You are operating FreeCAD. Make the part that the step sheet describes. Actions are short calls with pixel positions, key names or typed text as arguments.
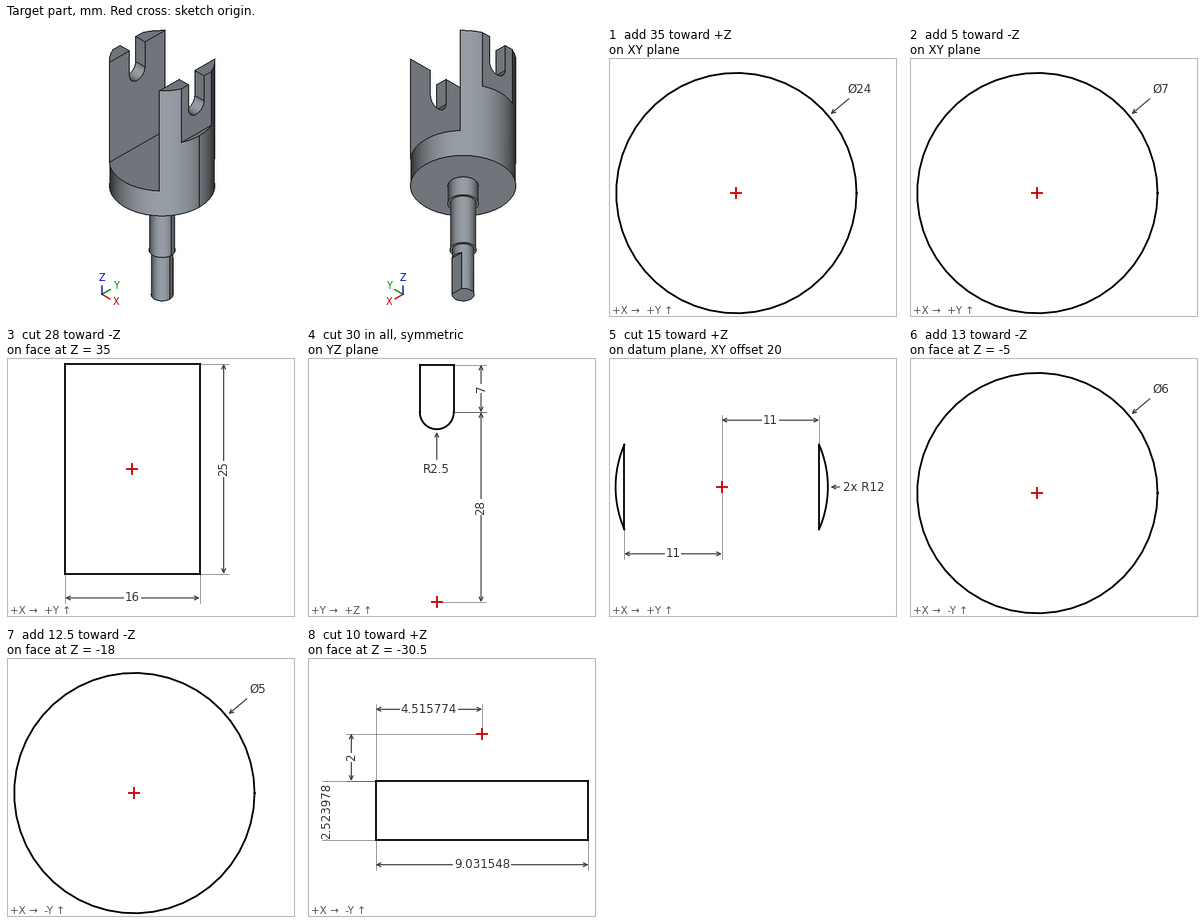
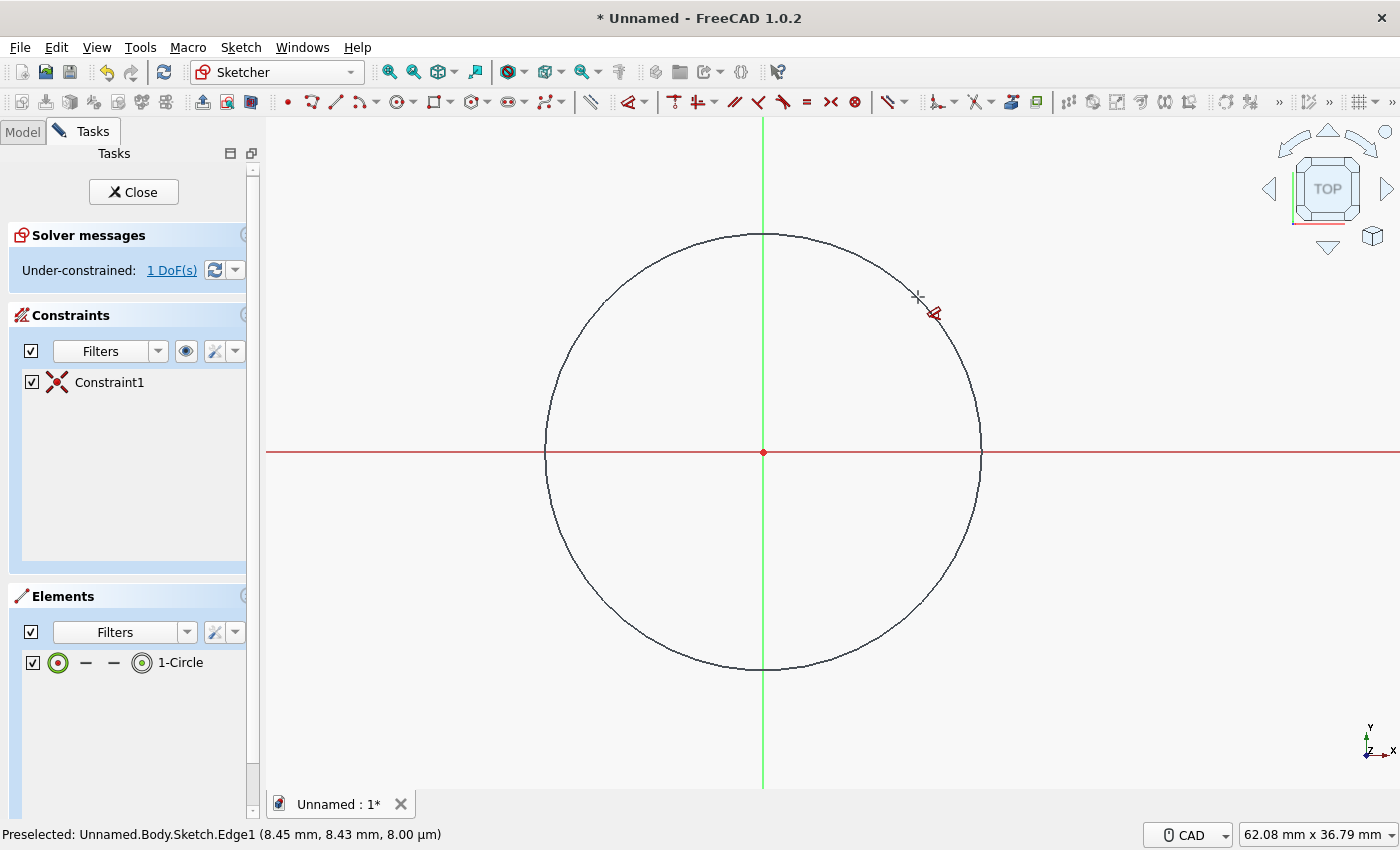
click(917, 297)
click(940, 274)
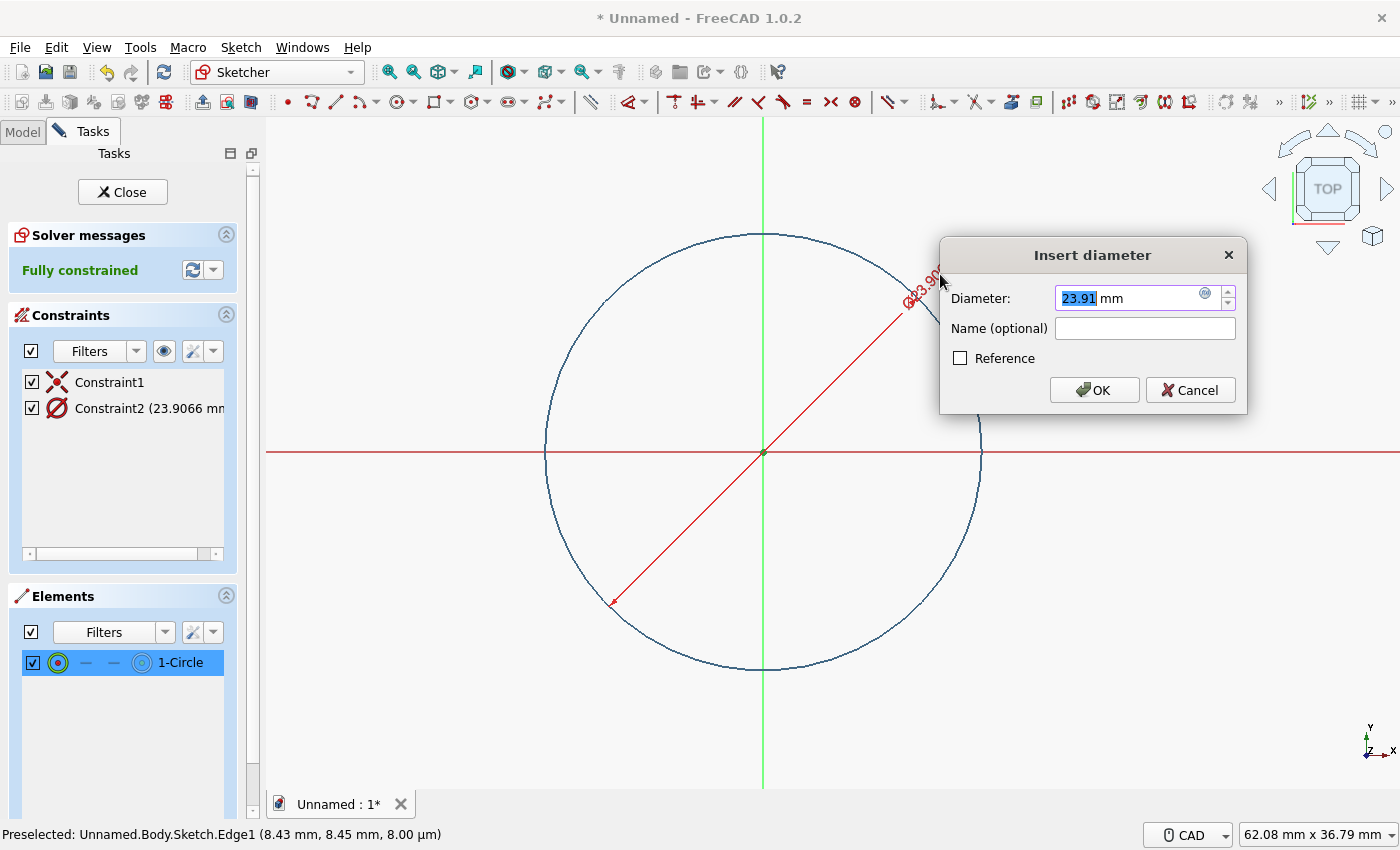
text(24)
key(Return)
key(Escape)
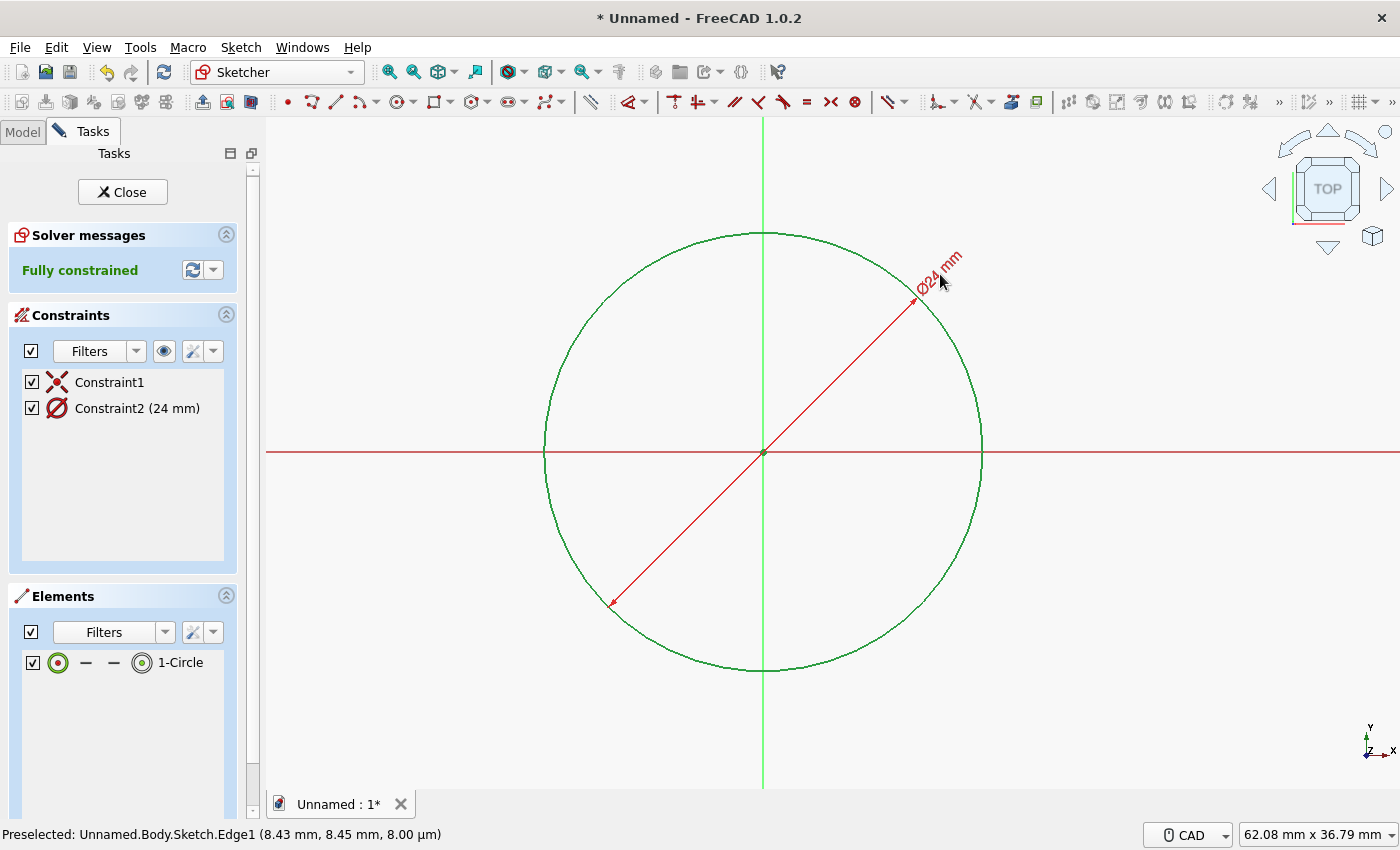
click(123, 192)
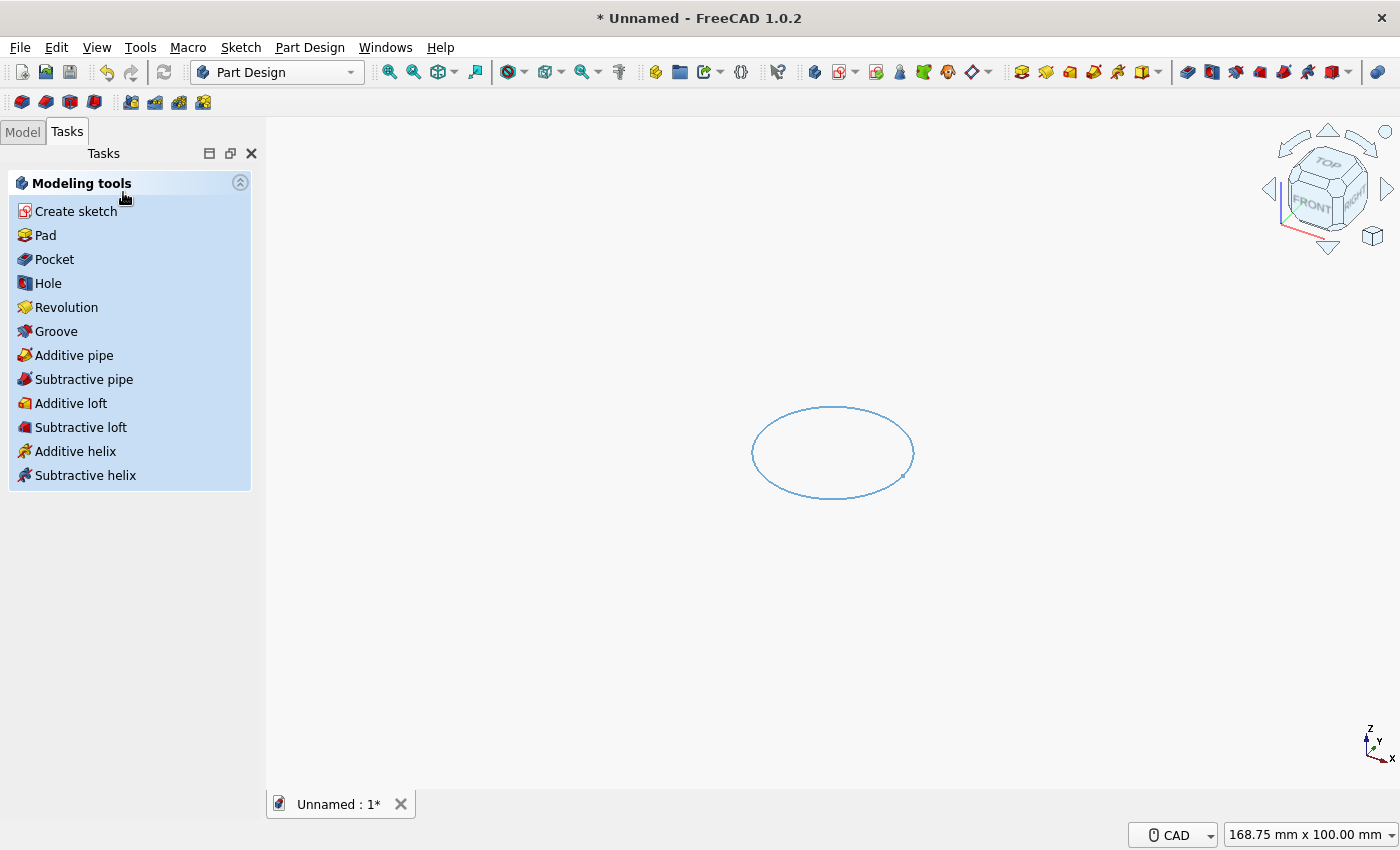
click(1022, 72)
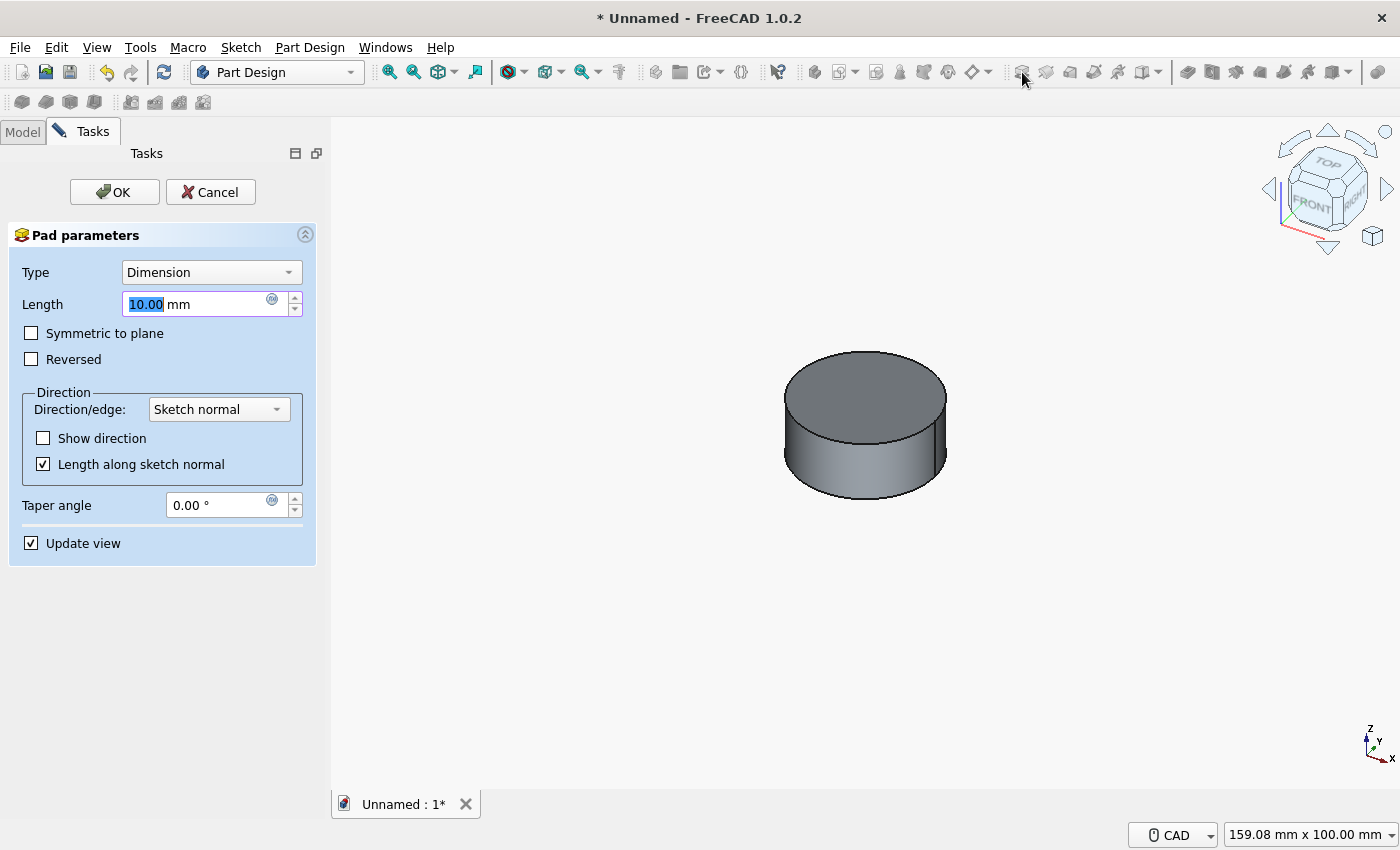
text(35)
key(Tab)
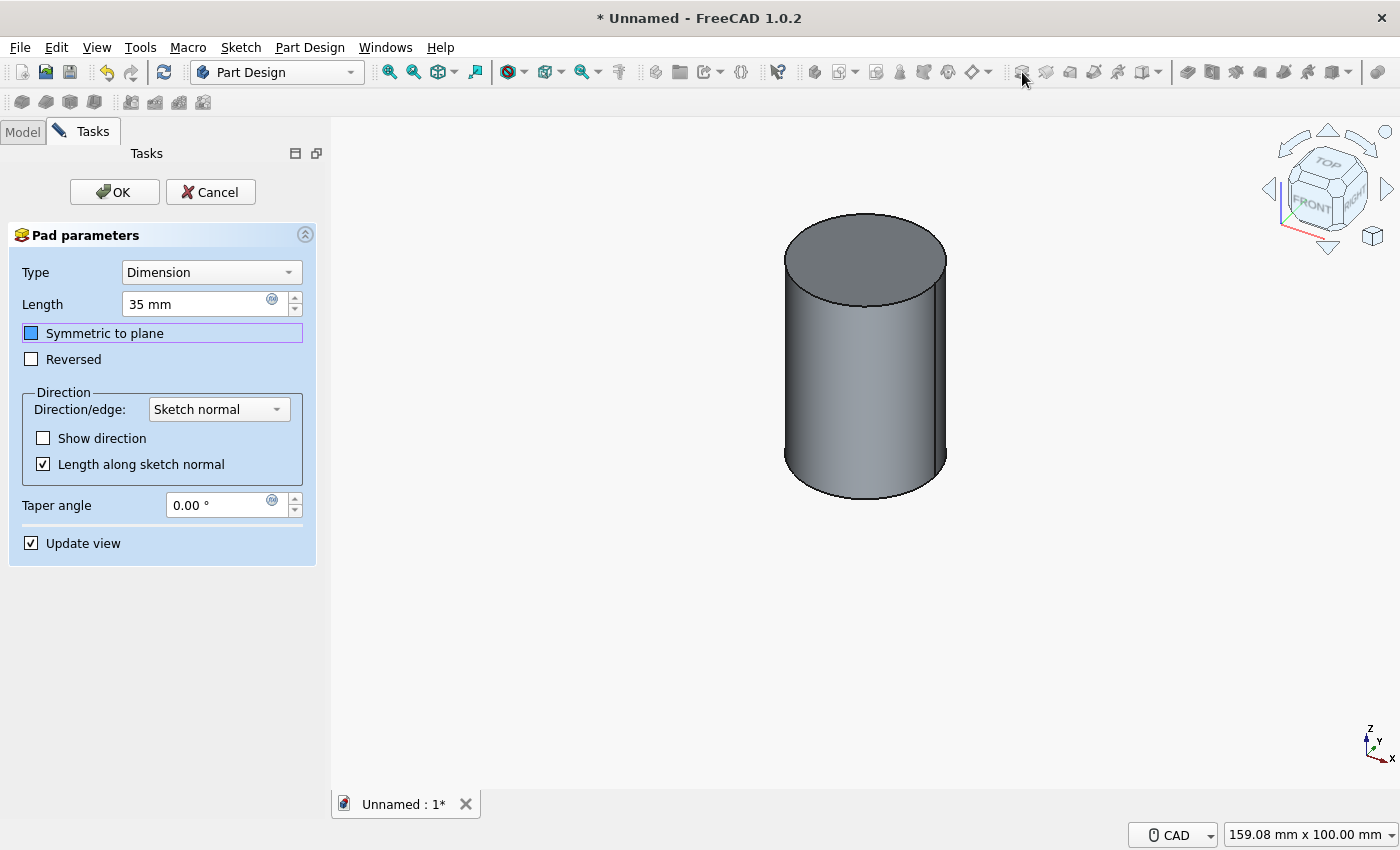
click(115, 192)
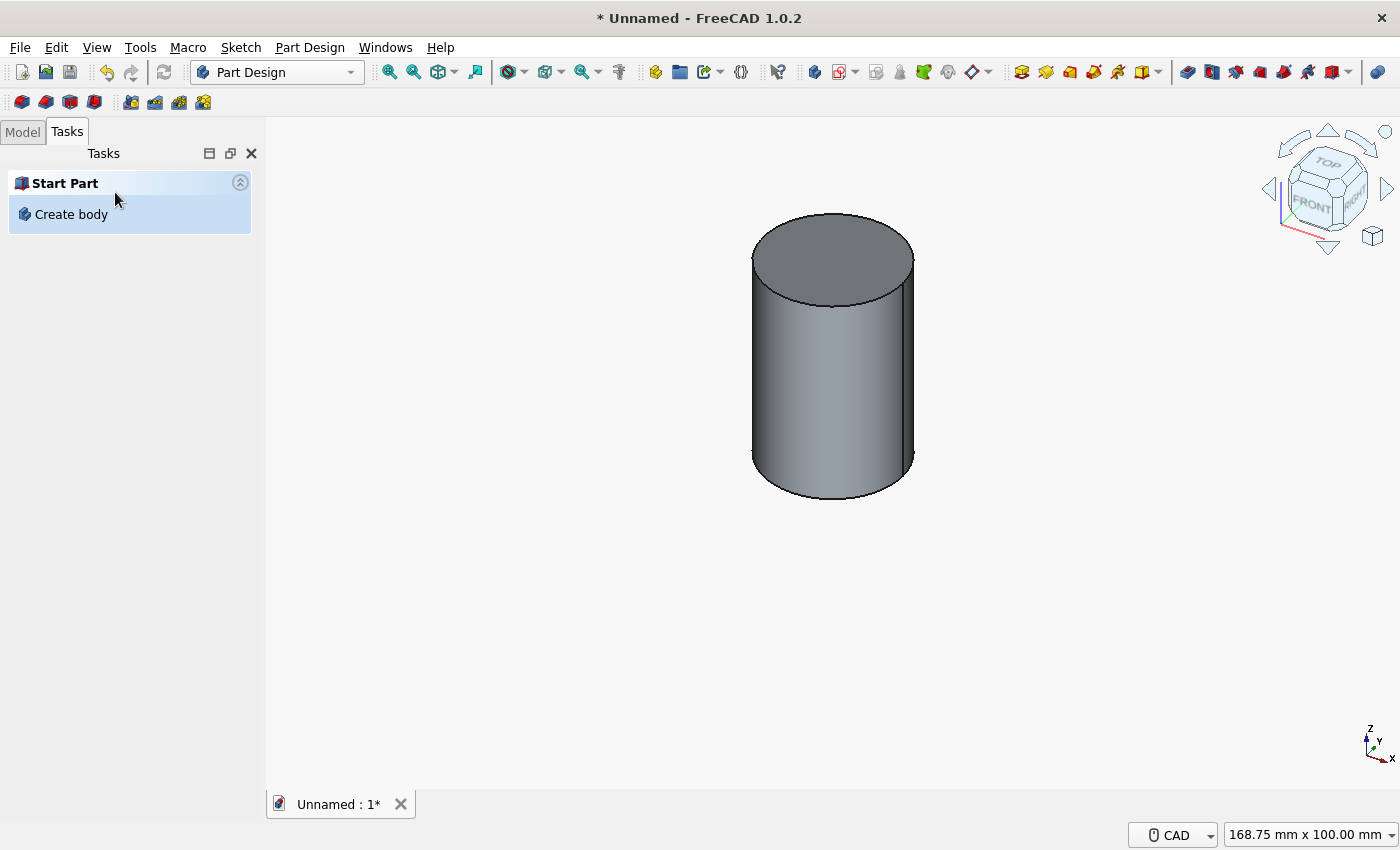
click(840, 72)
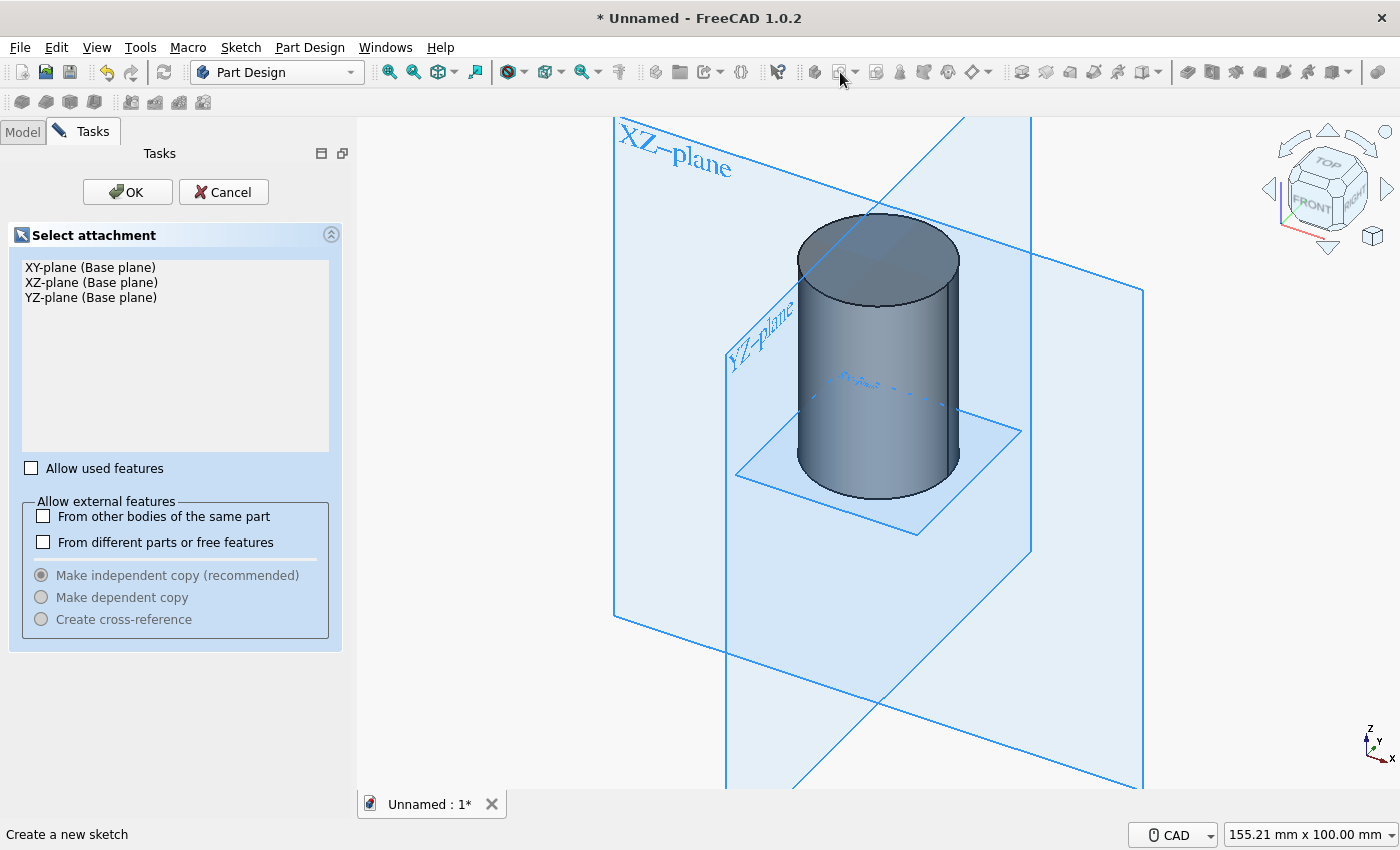
click(82, 268)